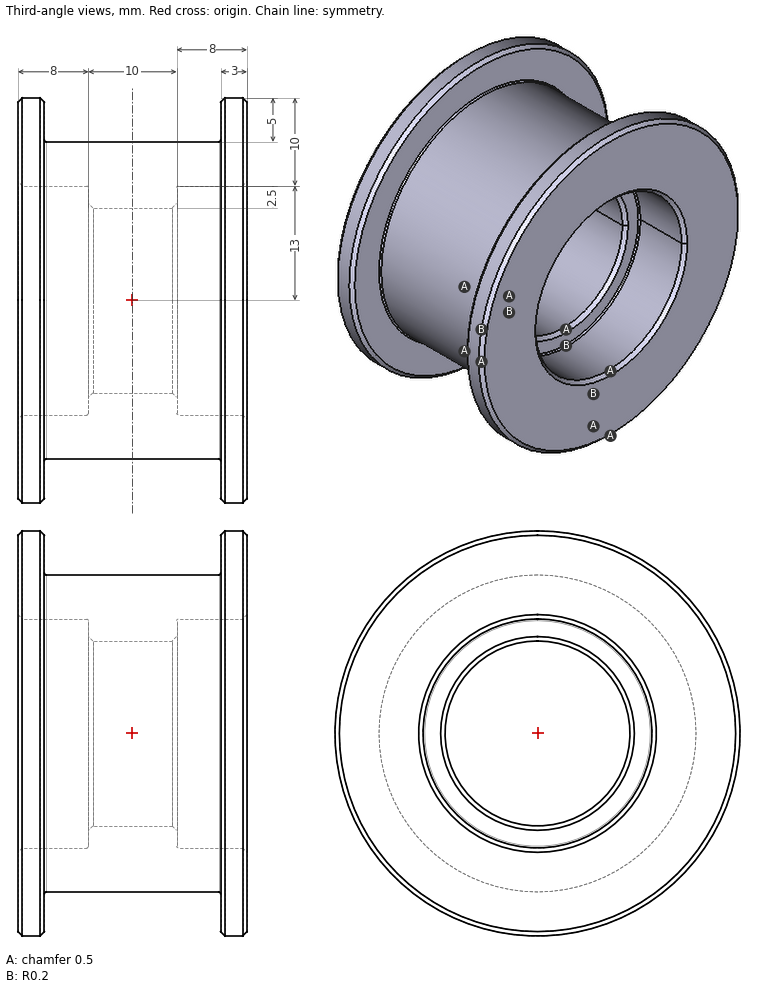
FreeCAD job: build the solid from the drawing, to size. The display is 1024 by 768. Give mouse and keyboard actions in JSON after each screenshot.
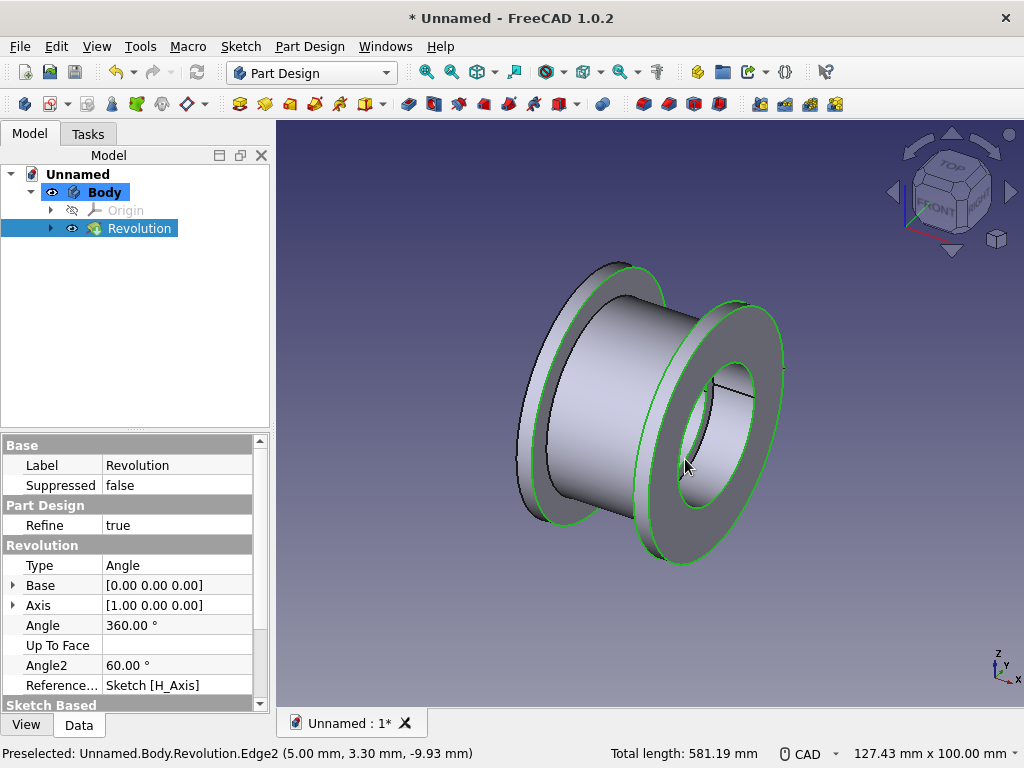
{"action": "key", "text": "0"}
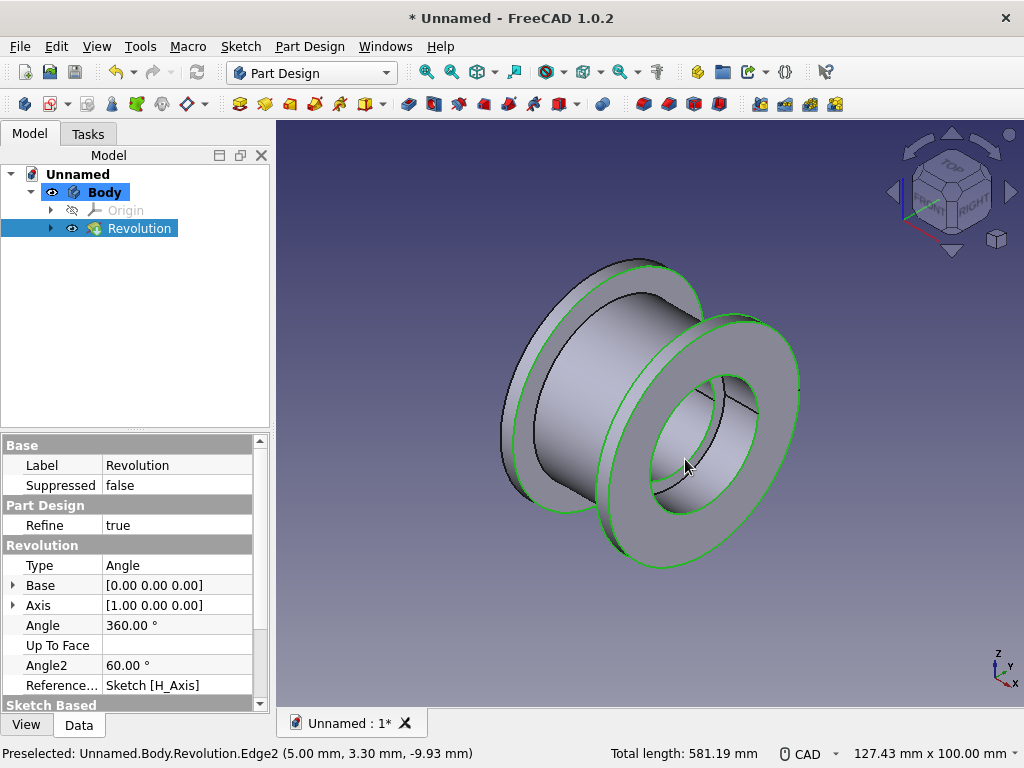
{"action": "left_click", "coordinate": [626, 259], "text": "ctrl"}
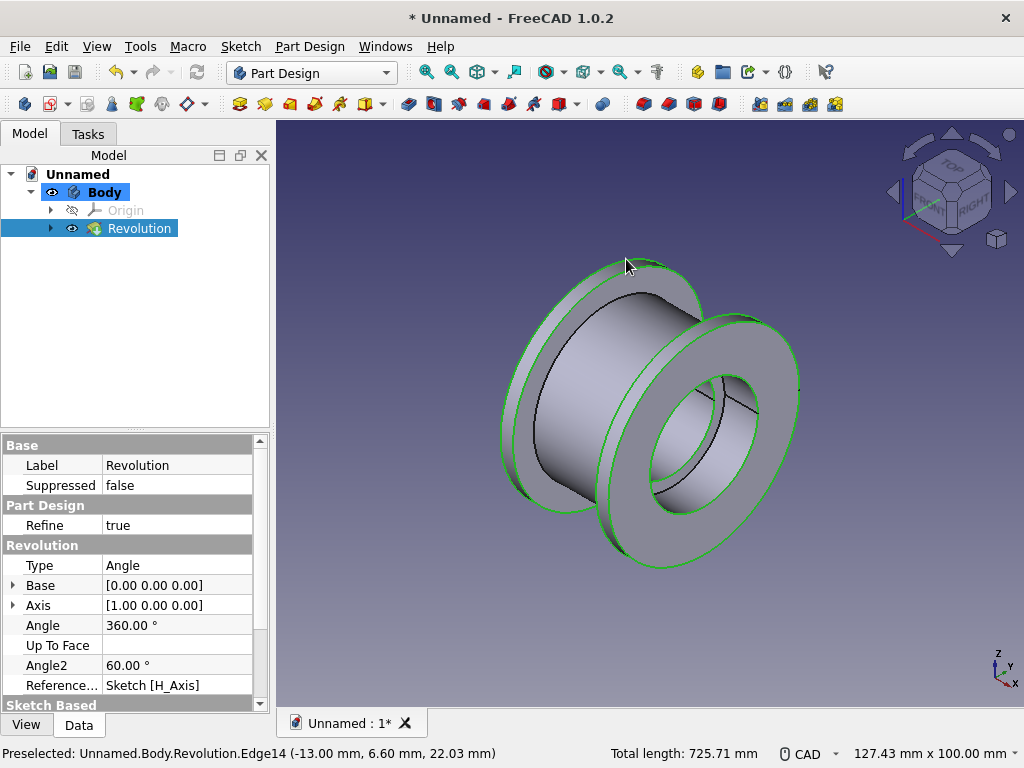
{"action": "key", "text": "2"}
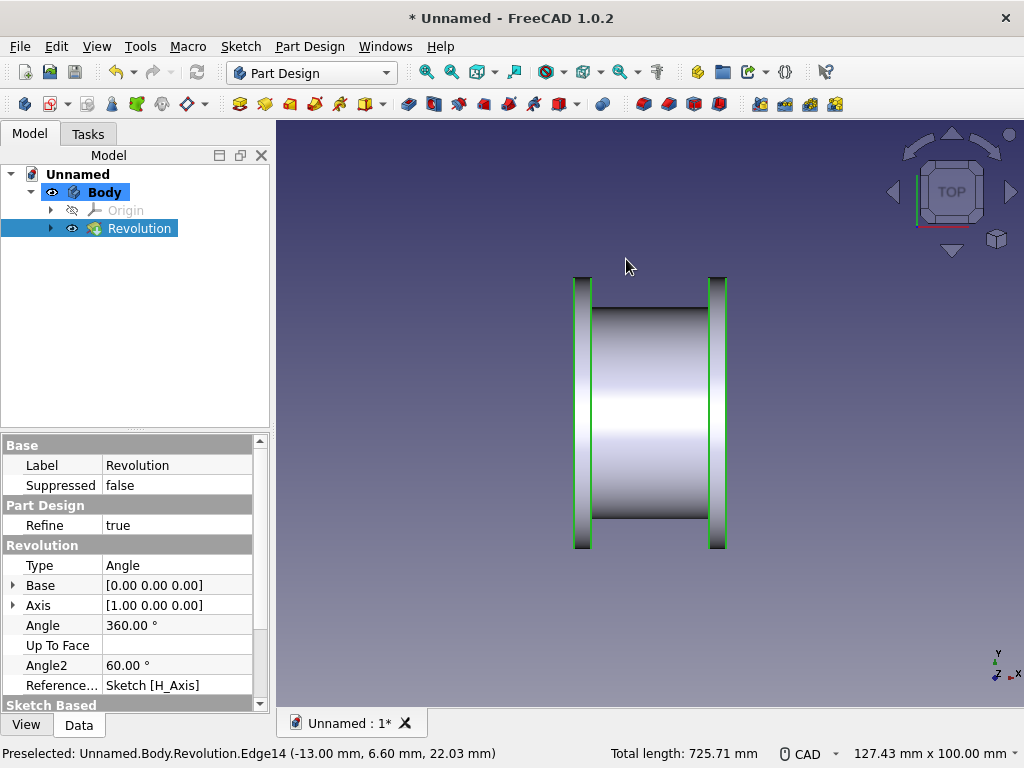
{"action": "key", "text": "1"}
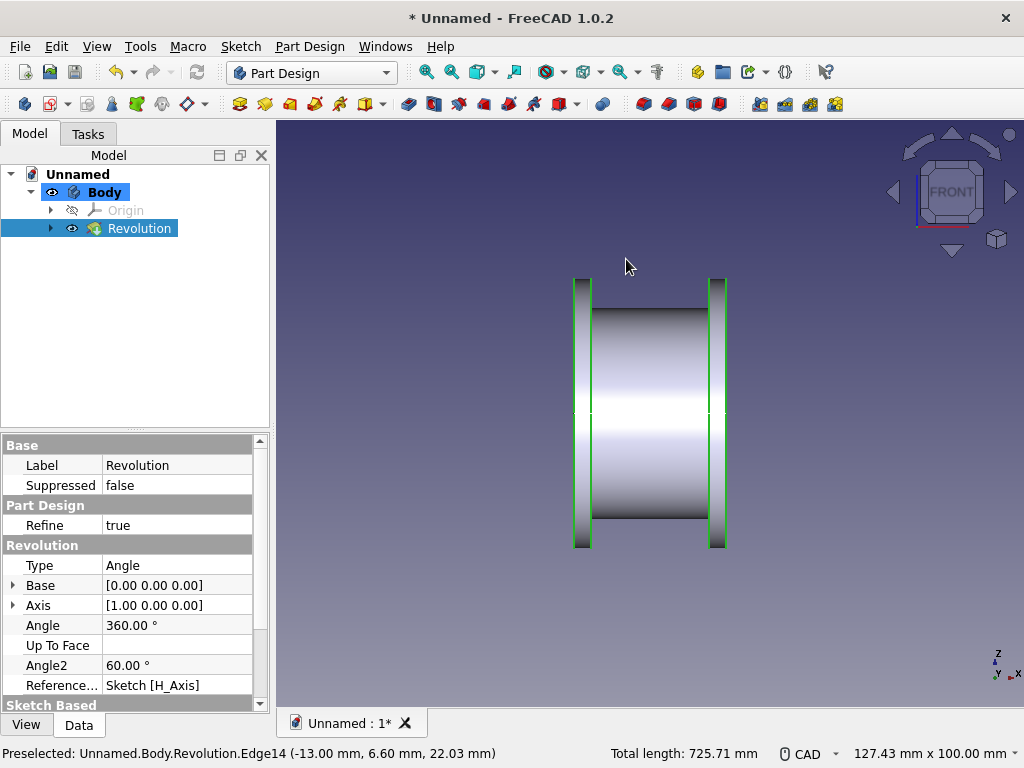
{"action": "key", "text": "3"}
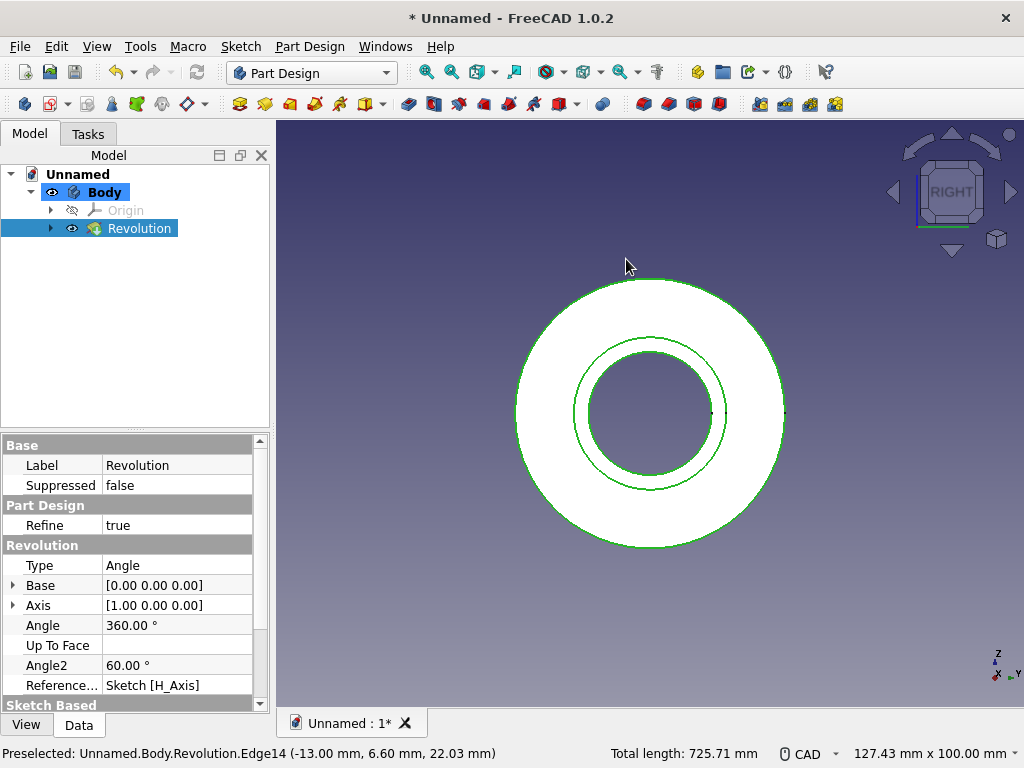
{"action": "key", "text": "5"}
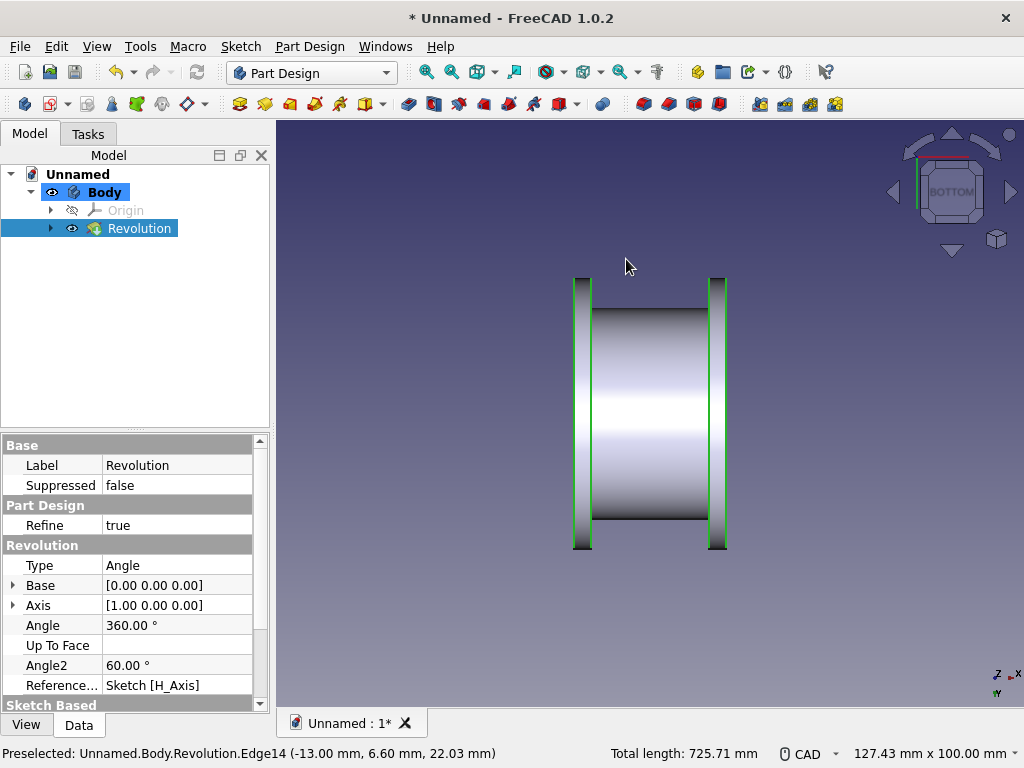
{"action": "key", "text": "4"}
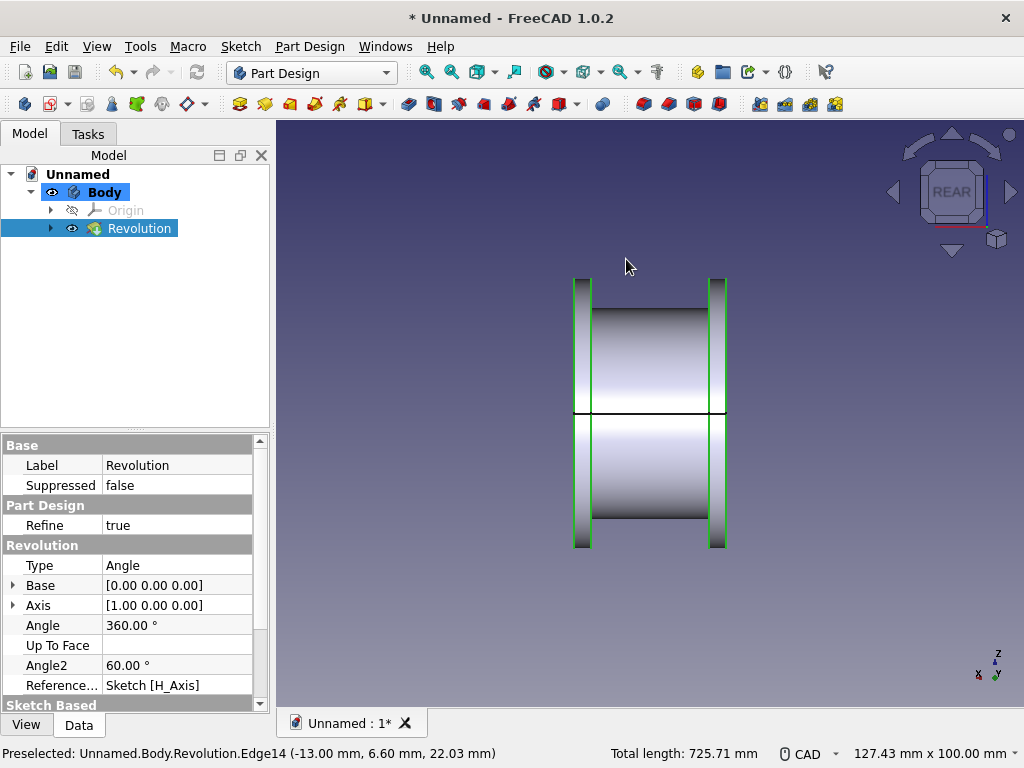
{"action": "key", "text": "6"}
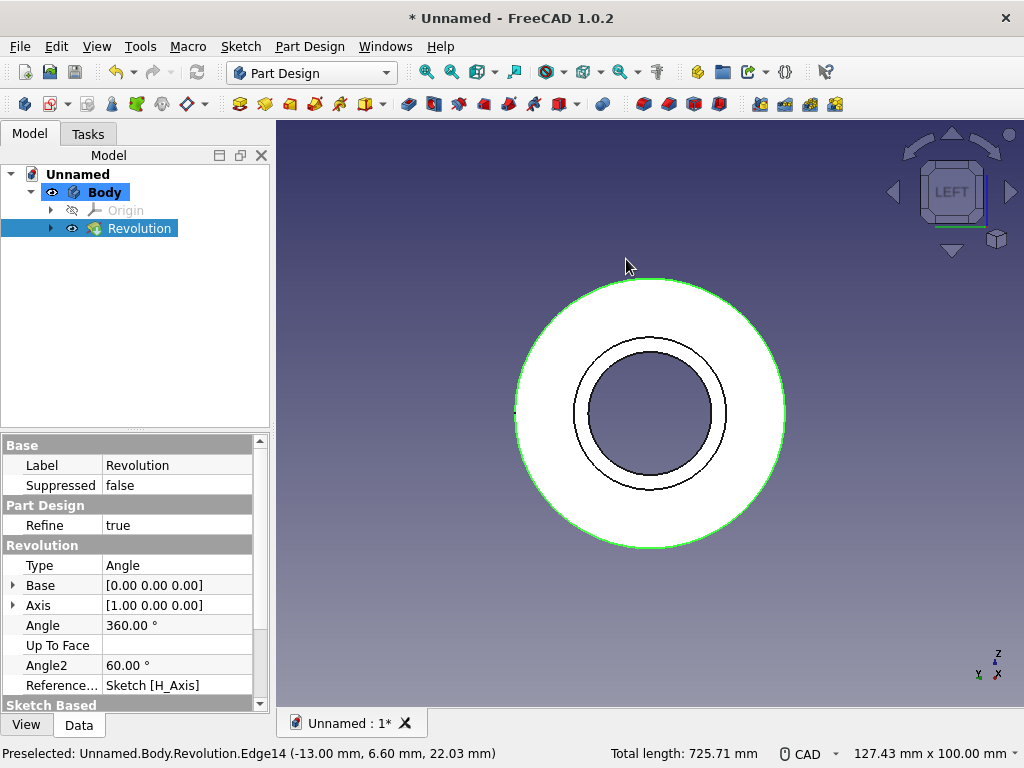
{"action": "left_click", "coordinate": [726, 412], "text": "ctrl"}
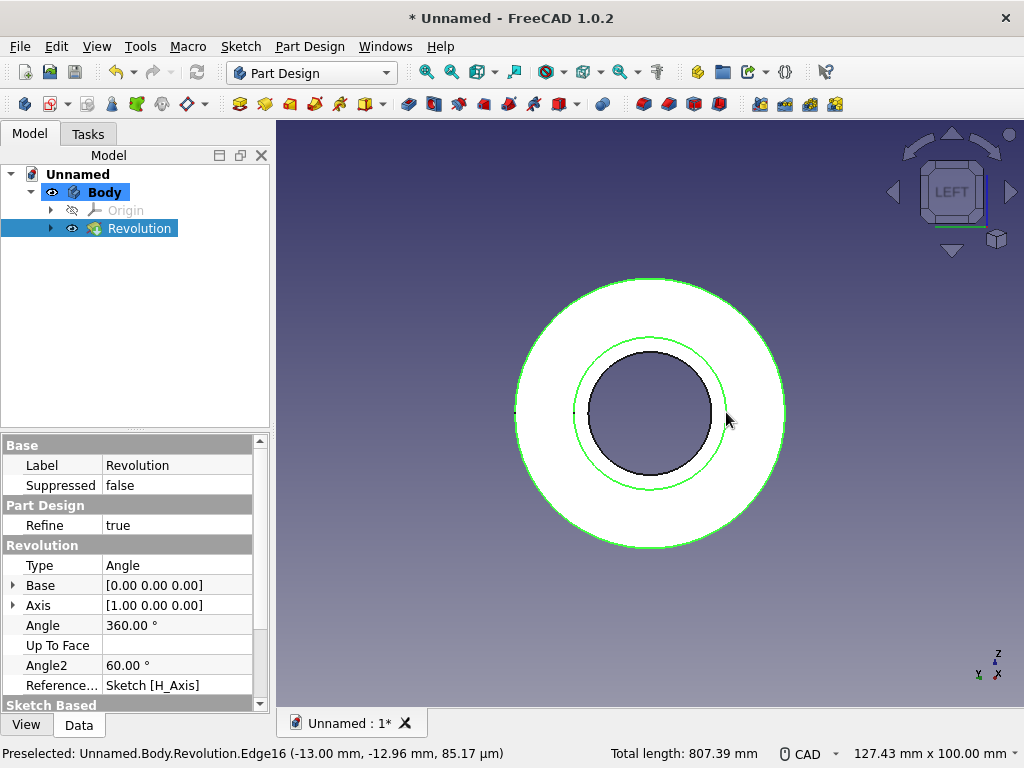
{"action": "left_click", "coordinate": [712, 412], "text": "ctrl"}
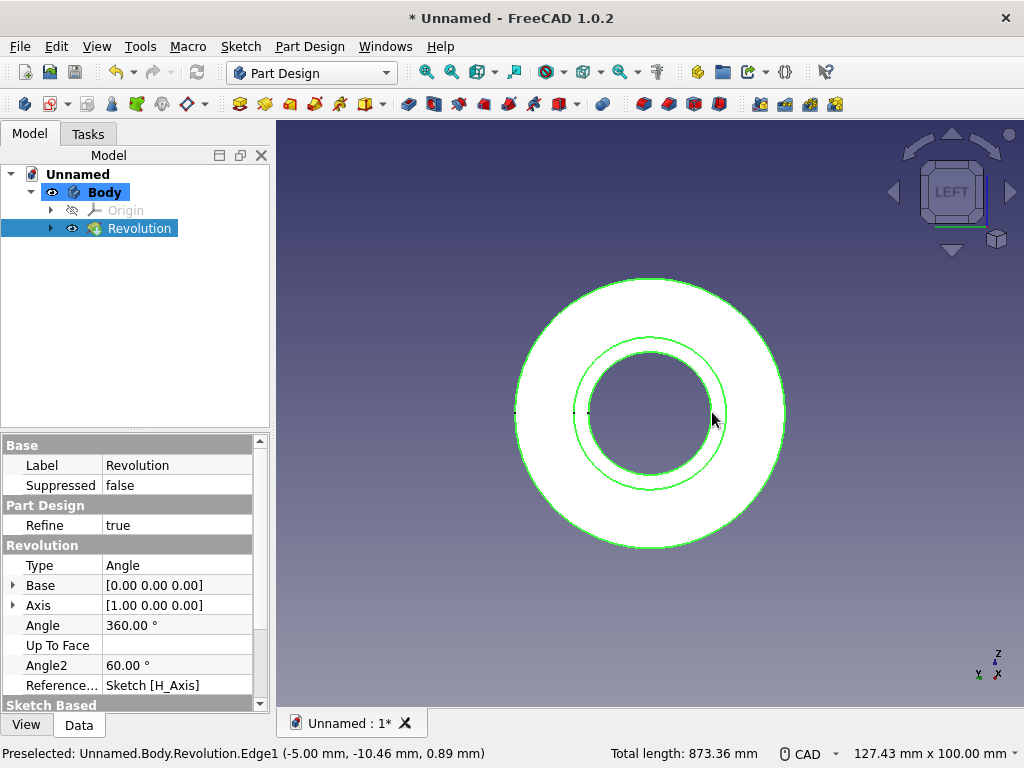
{"action": "left_click", "coordinate": [669, 104]}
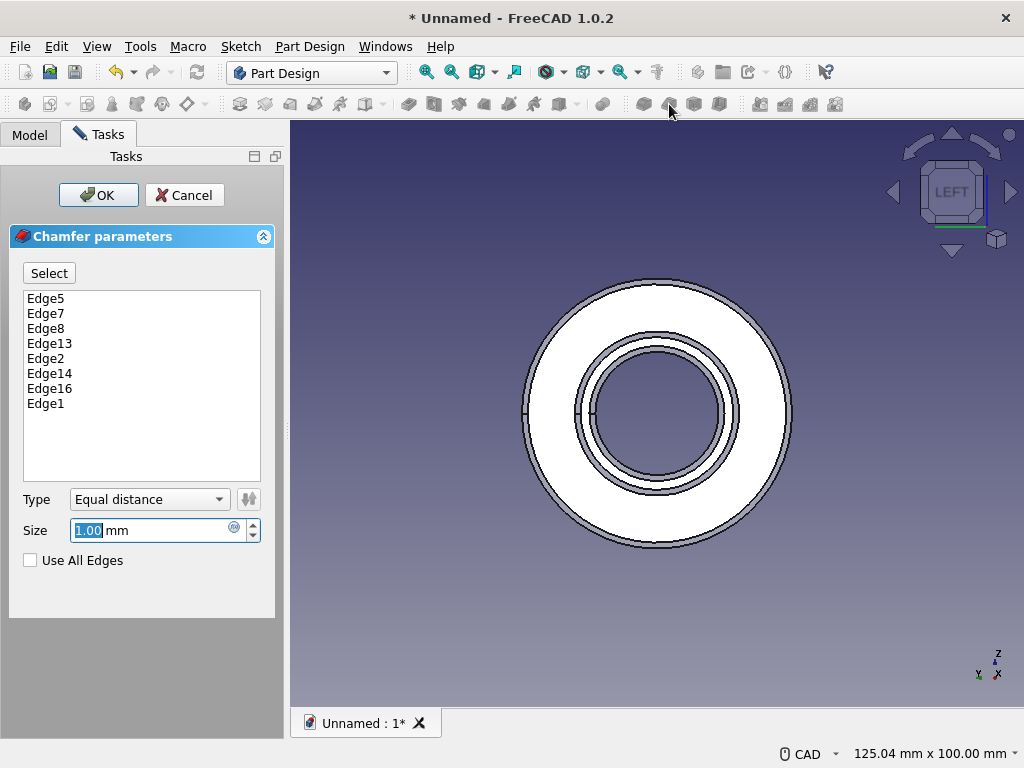
{"action": "type", "text": "0.5"}
{"action": "key", "text": "Tab"}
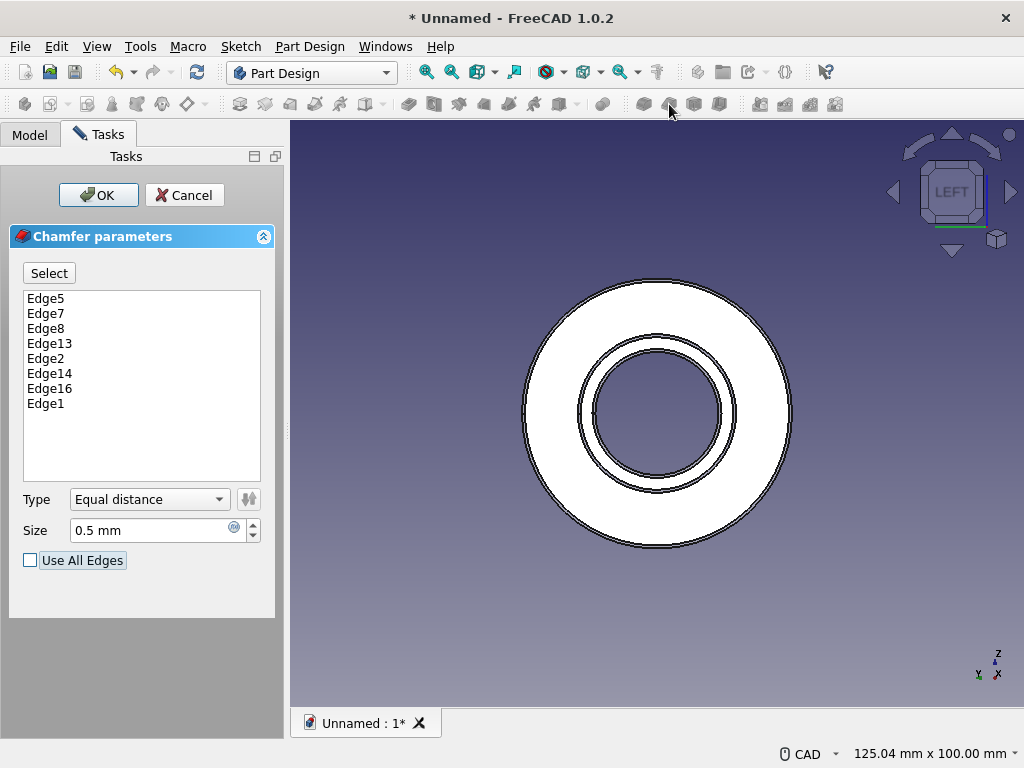
{"action": "left_click", "coordinate": [99, 195]}